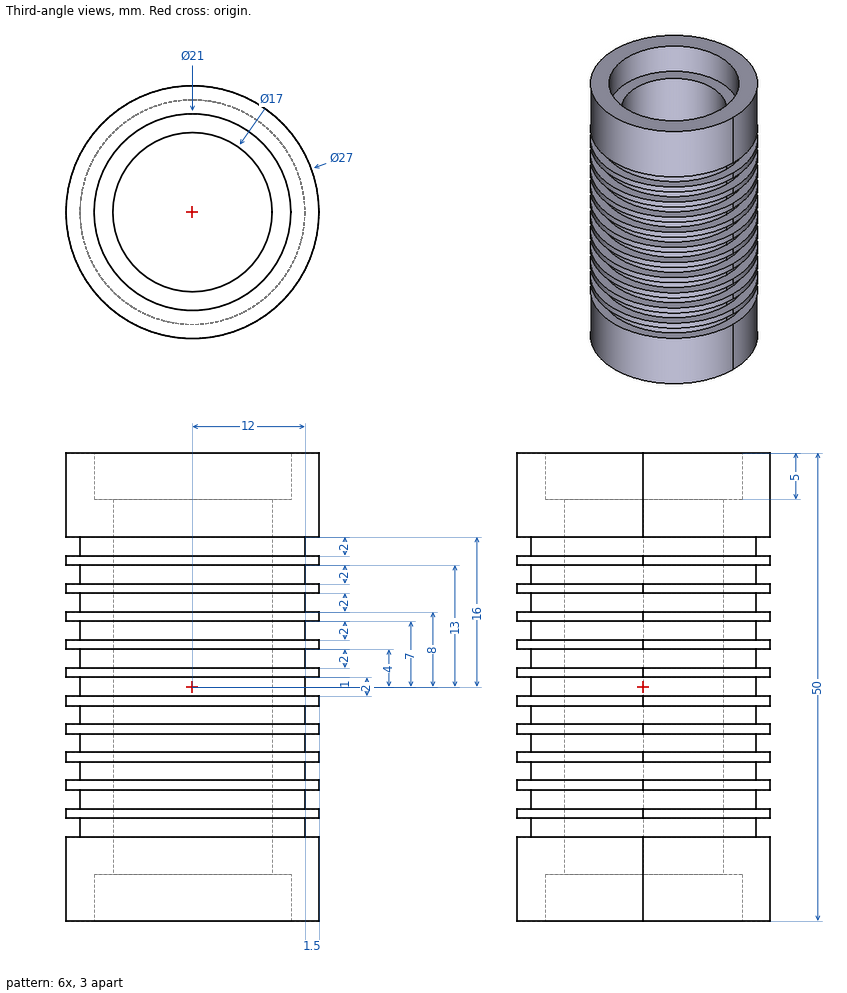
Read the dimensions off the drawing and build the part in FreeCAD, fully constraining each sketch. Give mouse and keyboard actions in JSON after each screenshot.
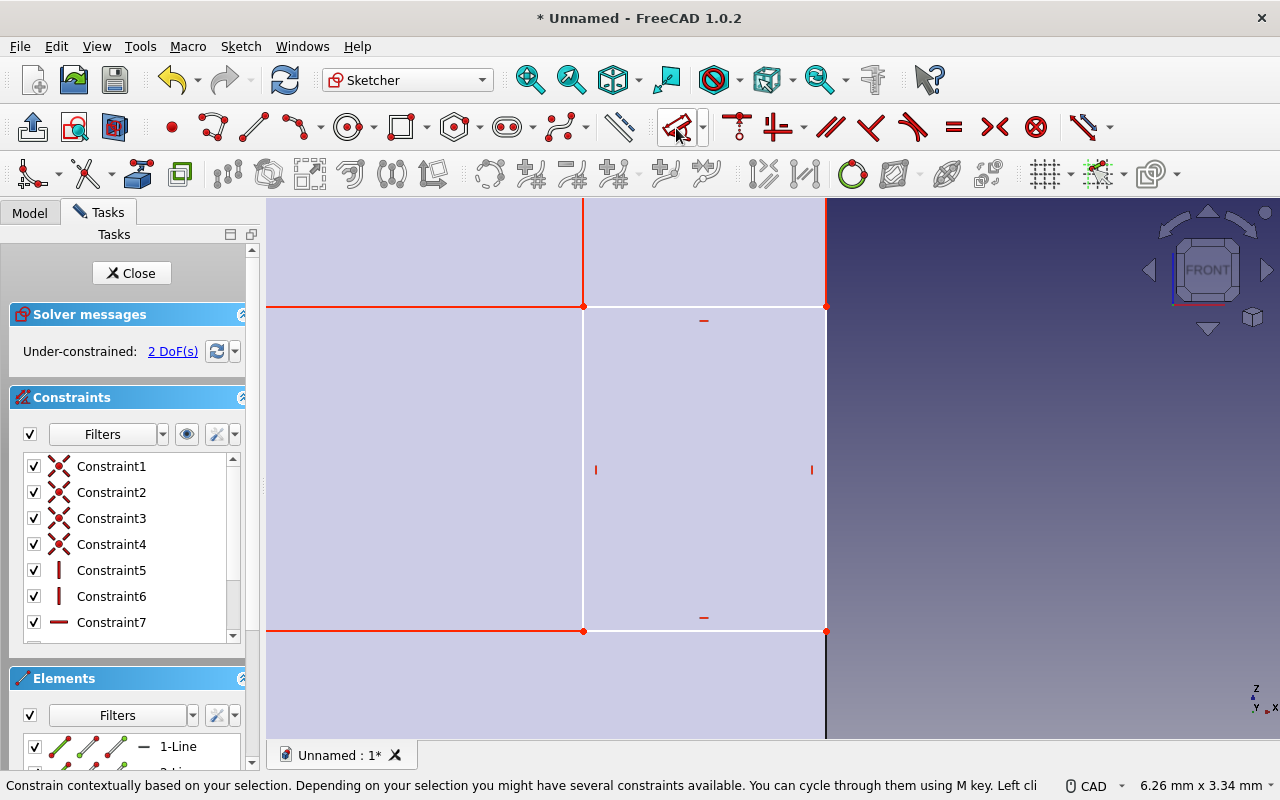
{"action": "left_click", "coordinate": [583, 631]}
{"action": "left_click", "coordinate": [617, 671]}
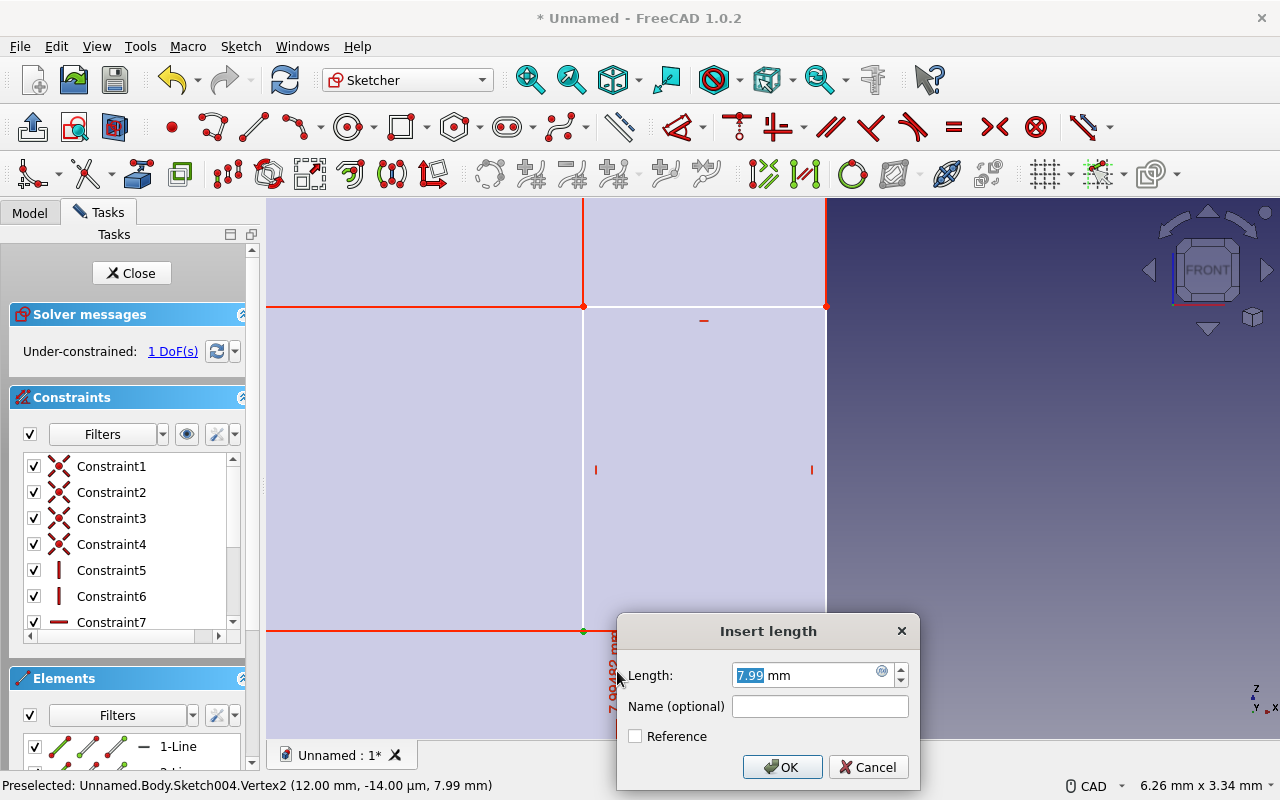
{"action": "type", "text": "8"}
{"action": "key", "text": "Return"}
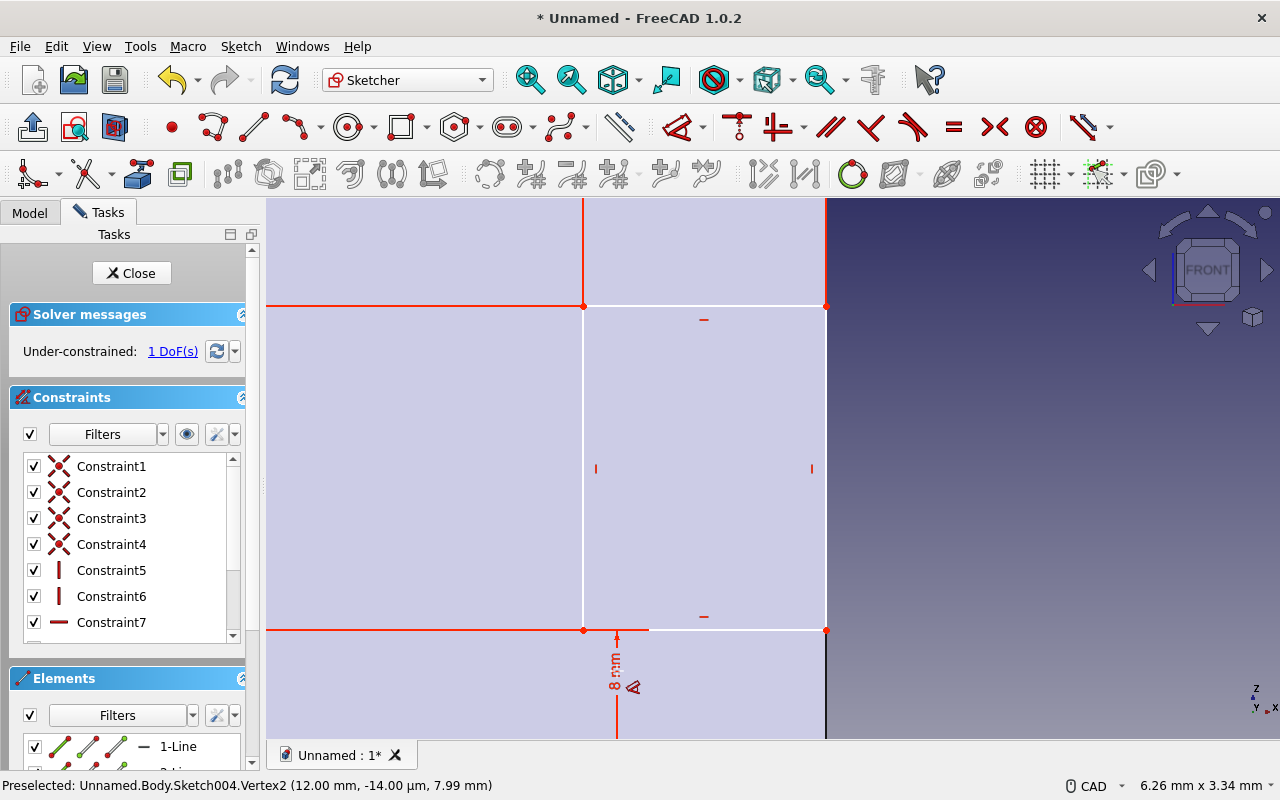
{"action": "left_click", "coordinate": [583, 306]}
{"action": "left_click", "coordinate": [438, 272]}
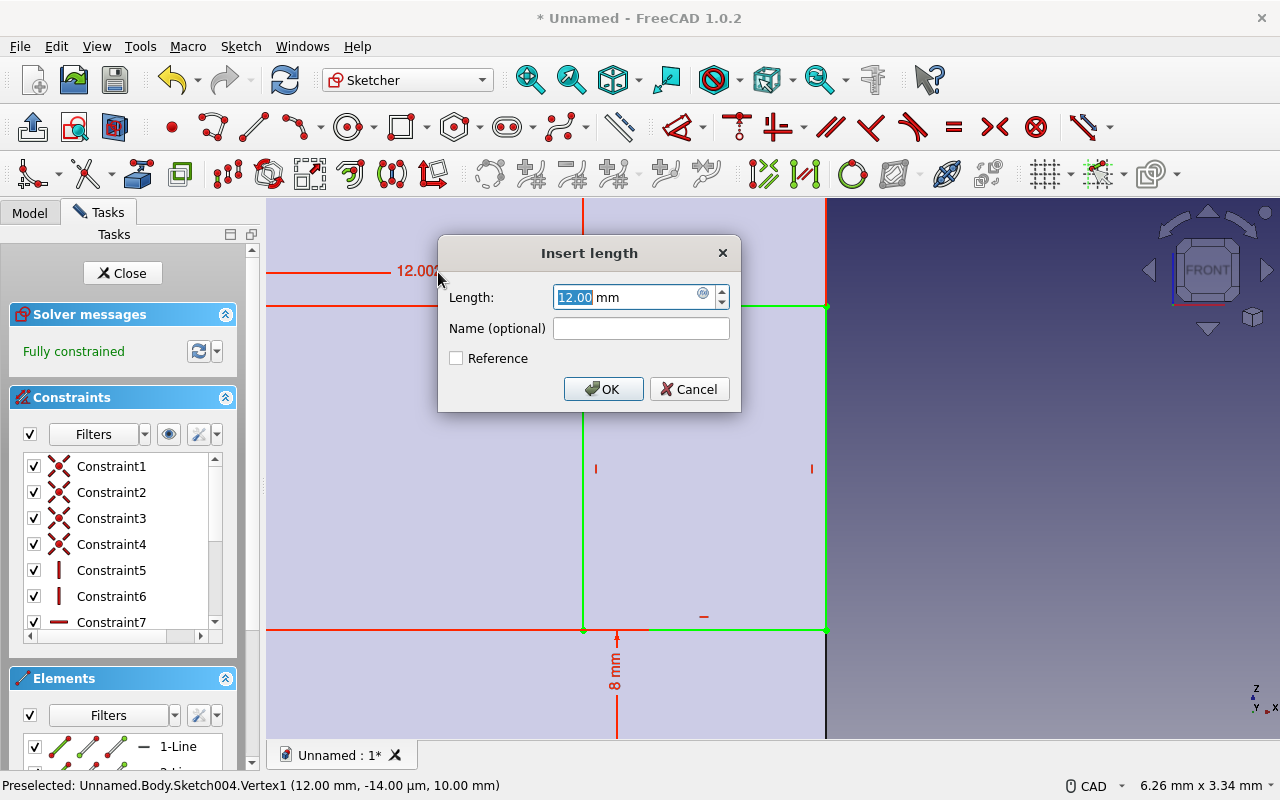
{"action": "type", "text": "12"}
{"action": "key", "text": "Return"}
{"action": "key", "text": "Escape"}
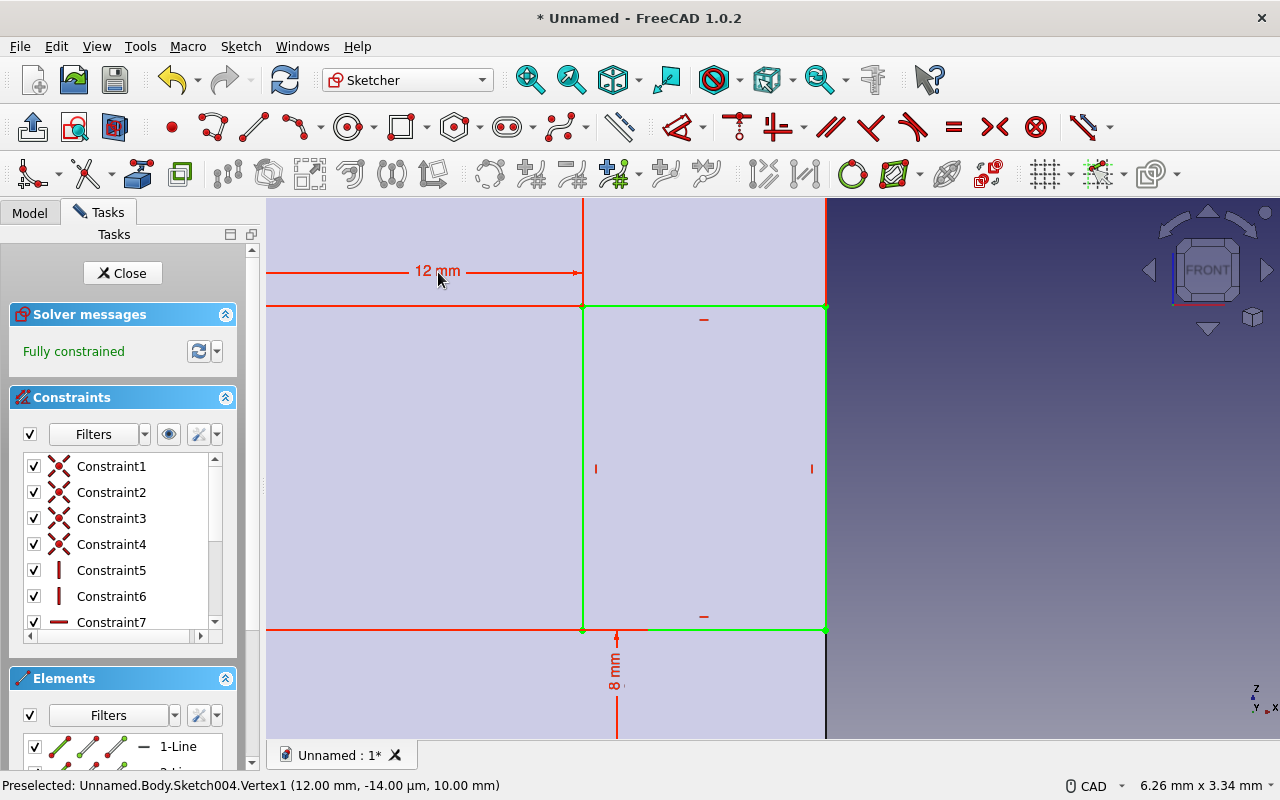
{"action": "left_click", "coordinate": [123, 273]}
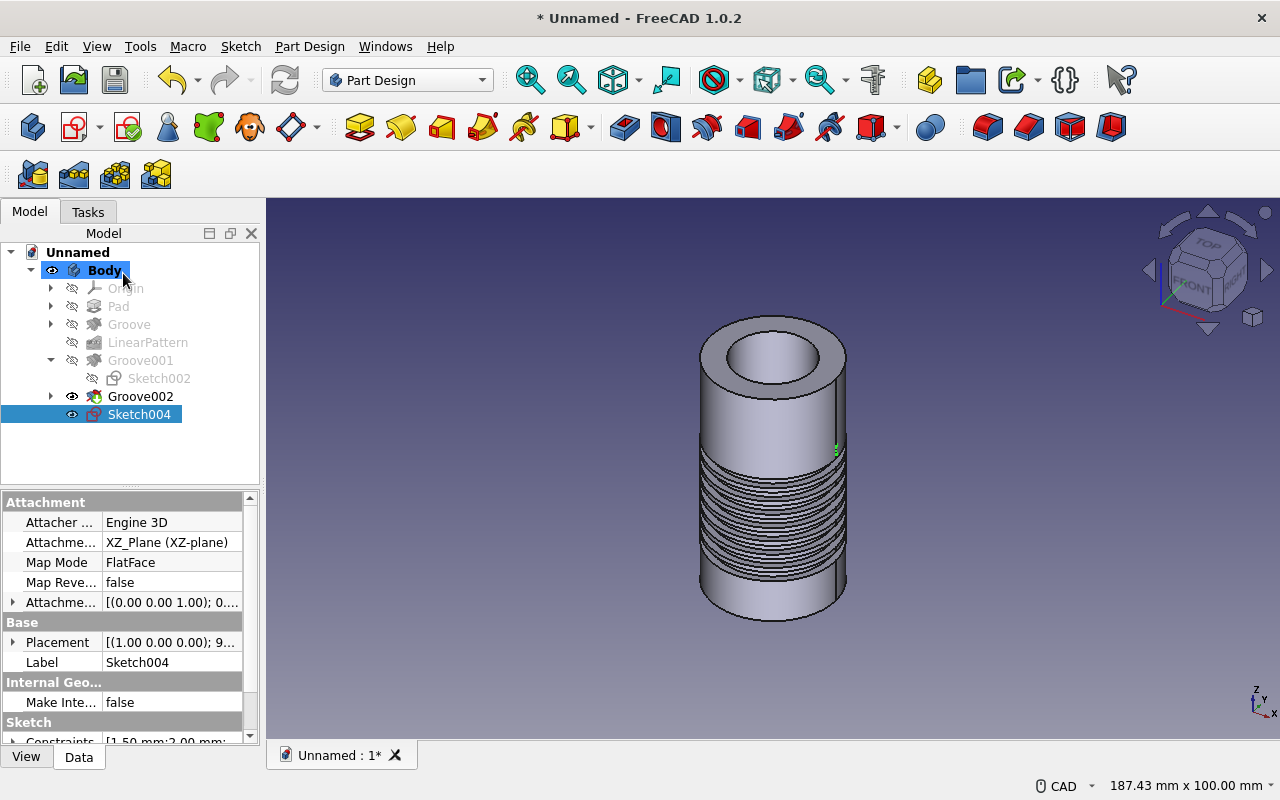
{"action": "left_click", "coordinate": [707, 128]}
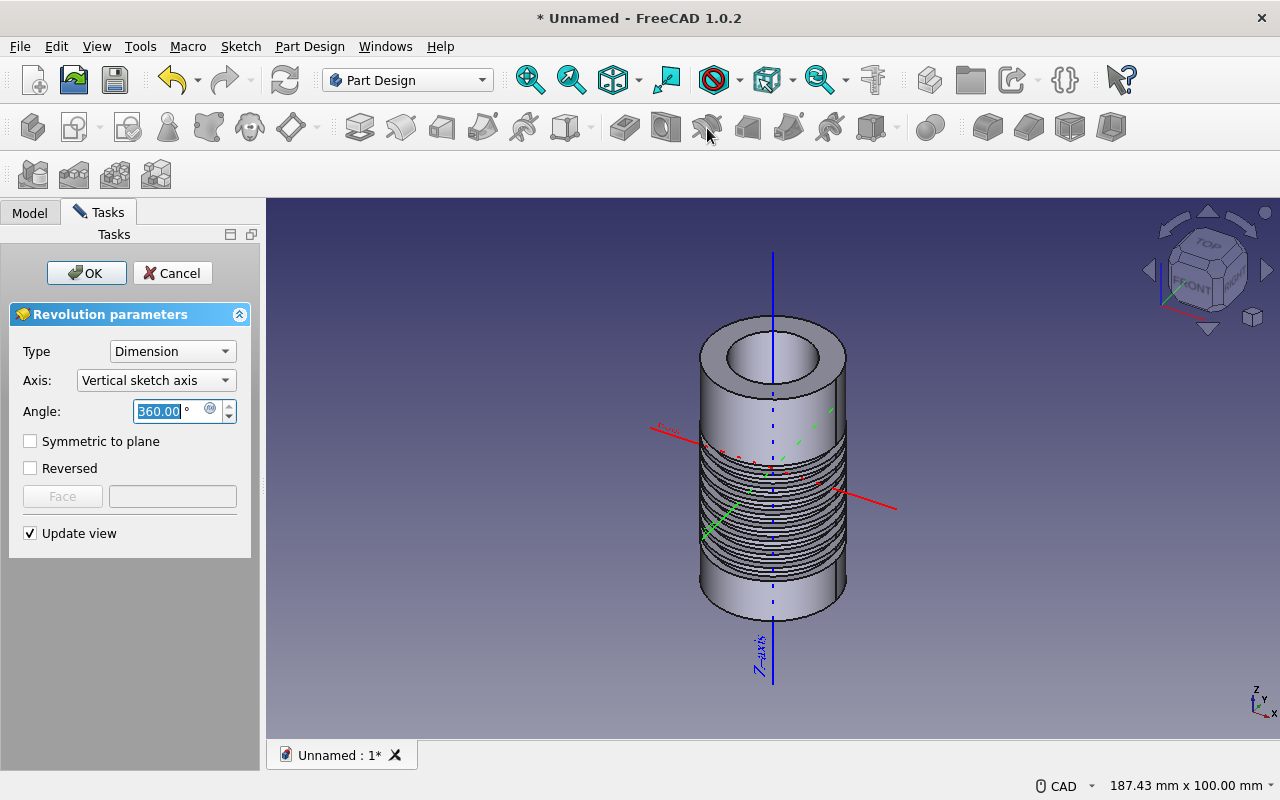
{"action": "left_click", "coordinate": [87, 273]}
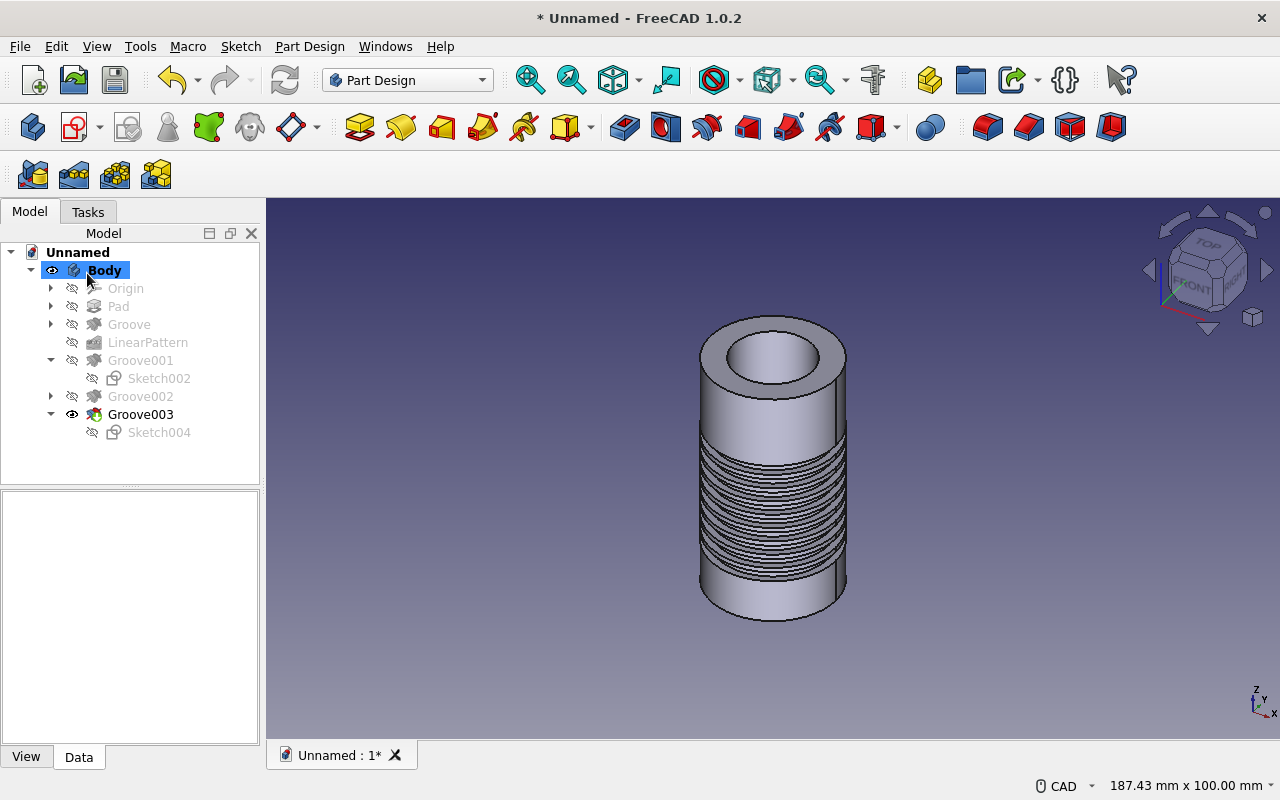
{"action": "left_click", "coordinate": [74, 128]}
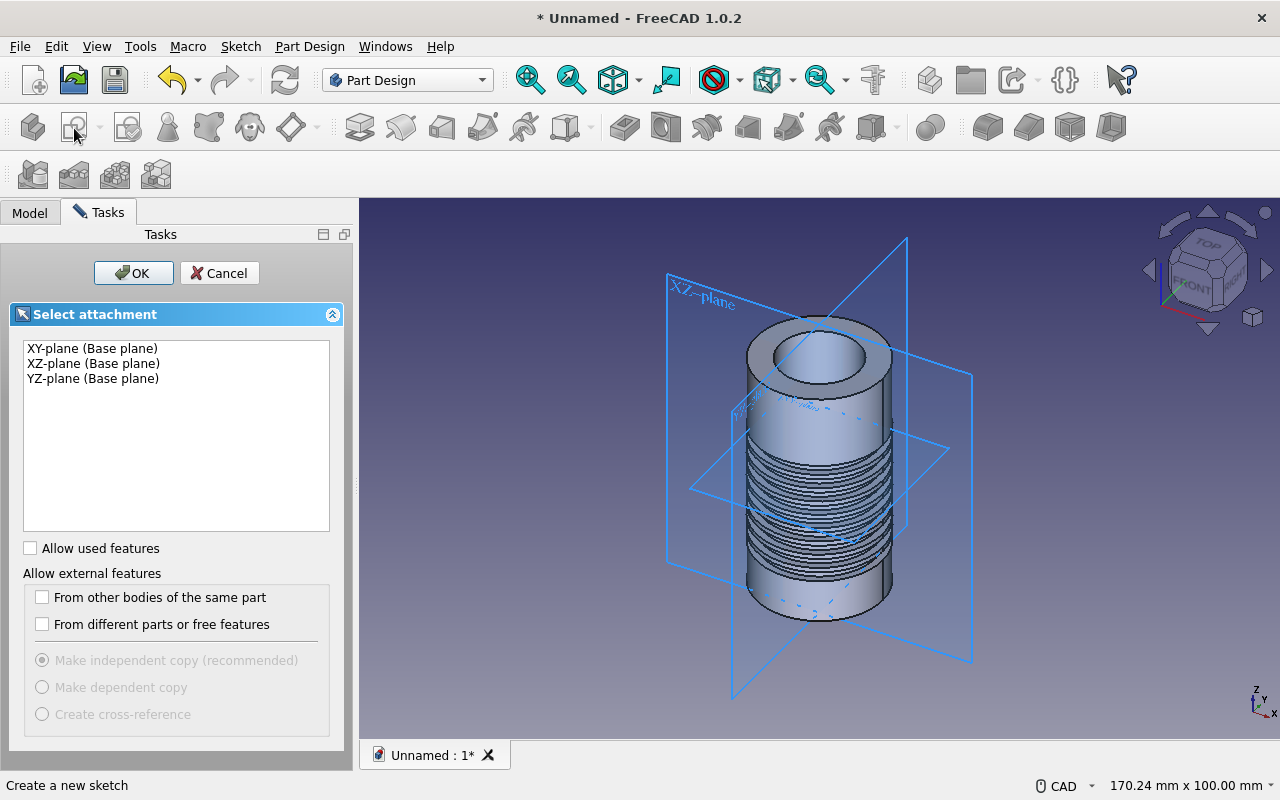
{"action": "left_click", "coordinate": [84, 364]}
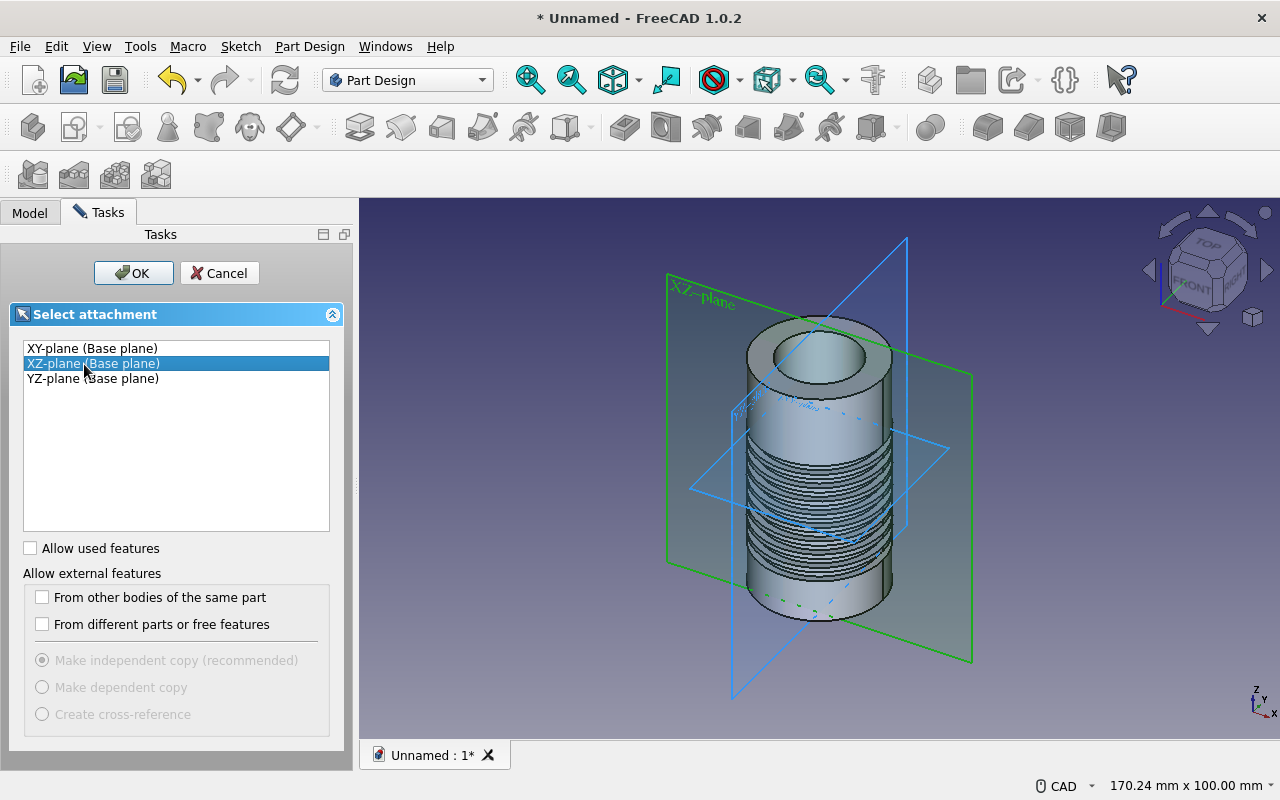
{"action": "left_click", "coordinate": [134, 273]}